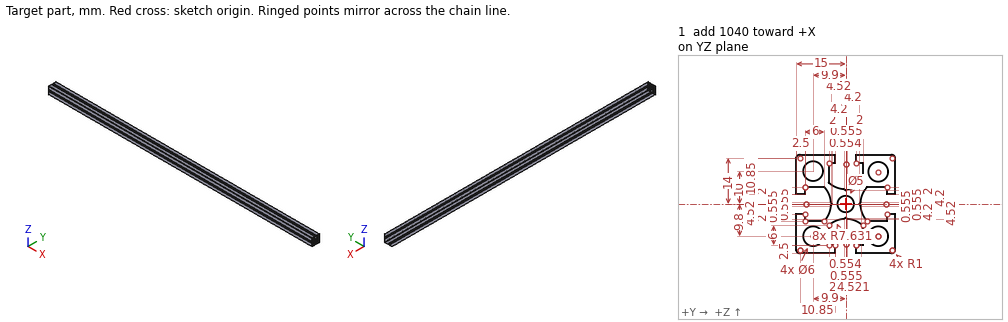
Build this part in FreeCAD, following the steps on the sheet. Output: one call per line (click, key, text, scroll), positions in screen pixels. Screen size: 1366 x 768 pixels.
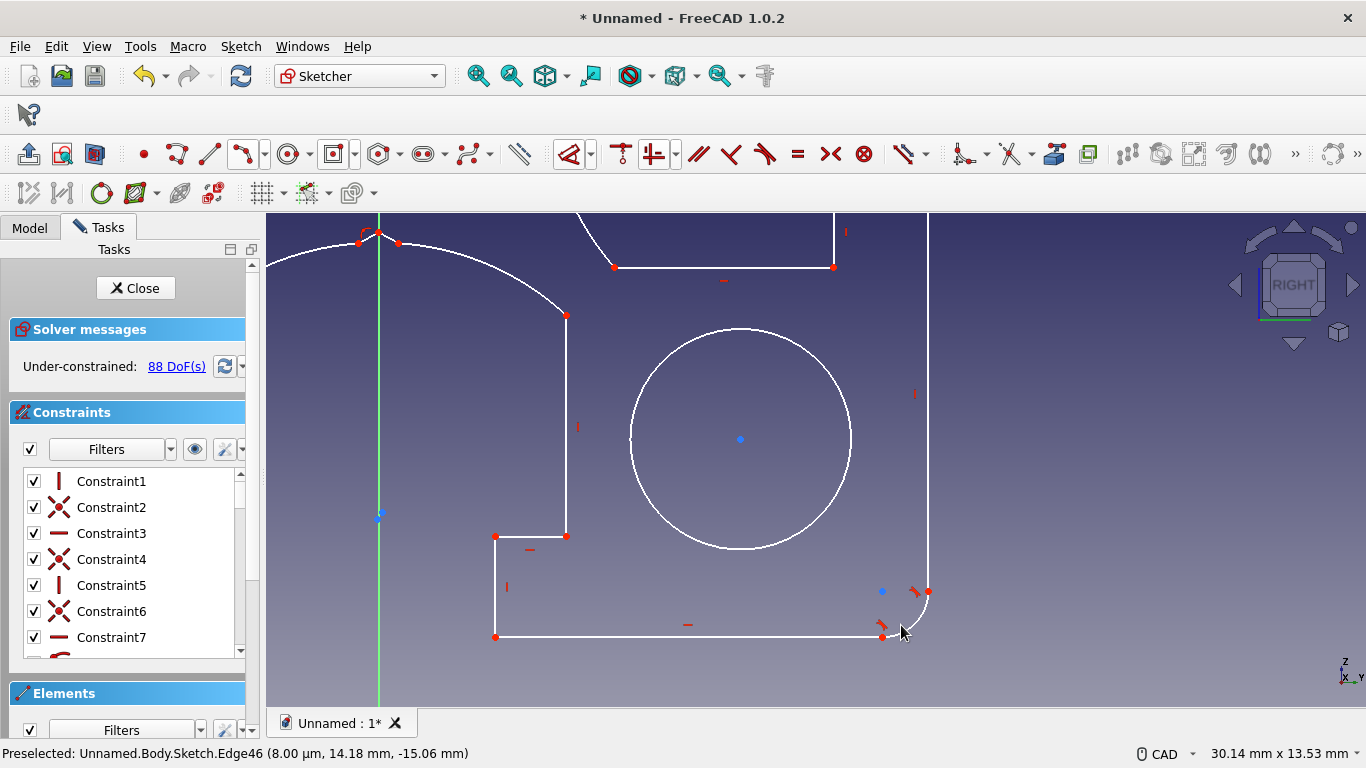
scroll(906, 625, down, 6)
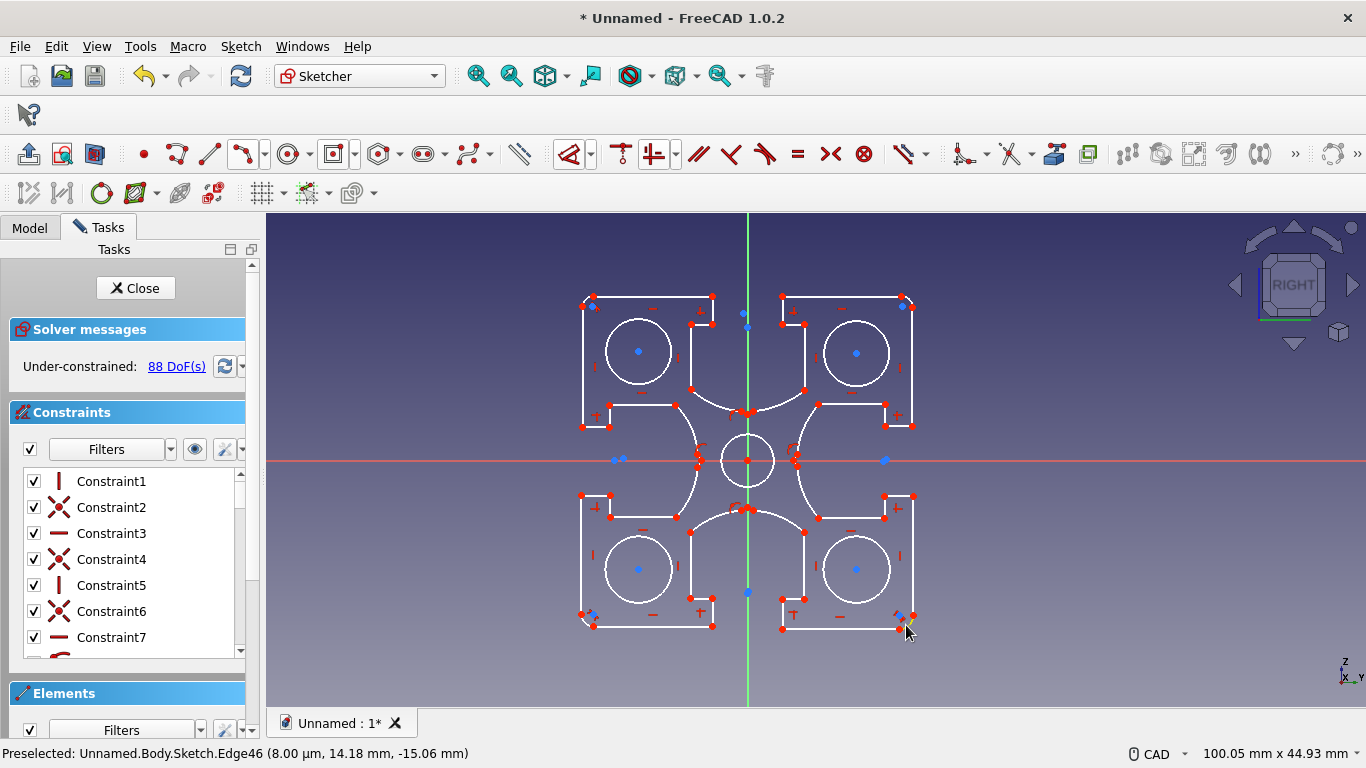
click(912, 391)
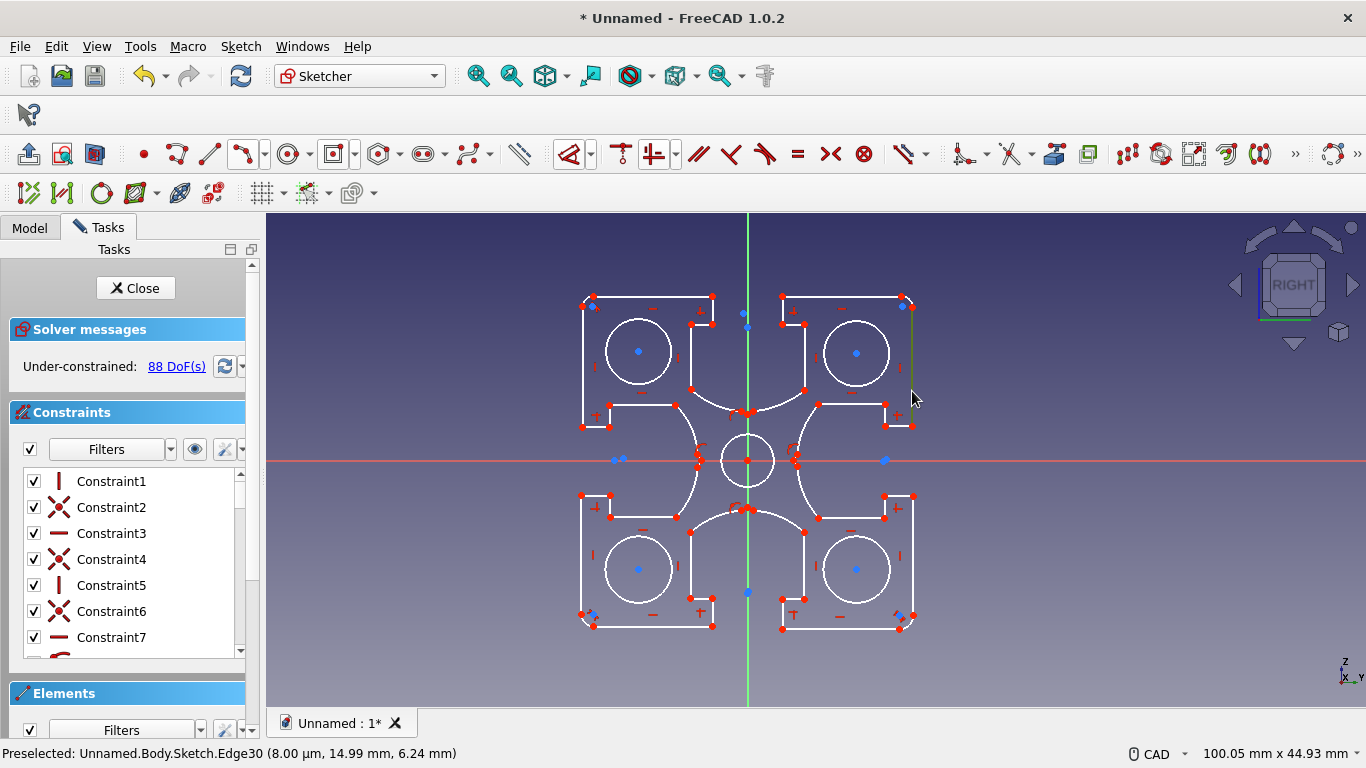
scroll(910, 300, up, 3)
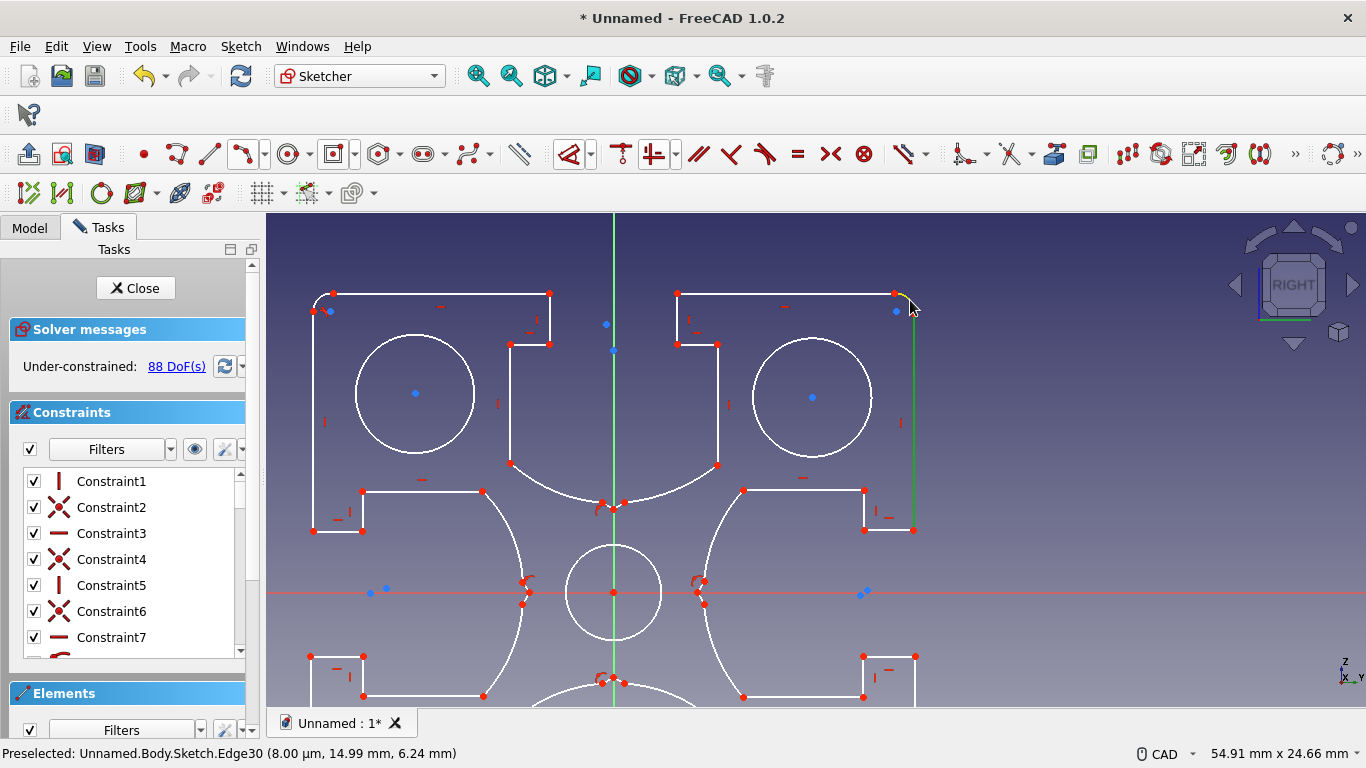
click(909, 299)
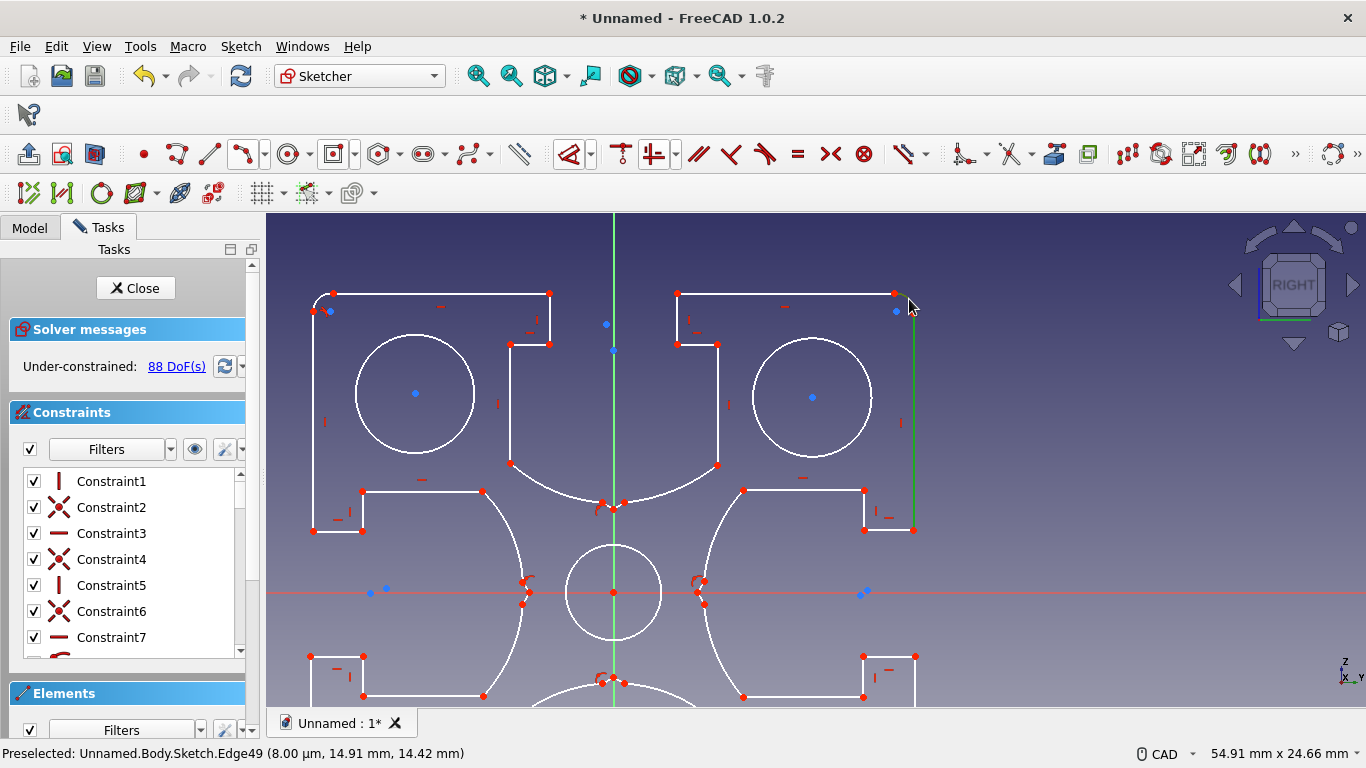
key(t)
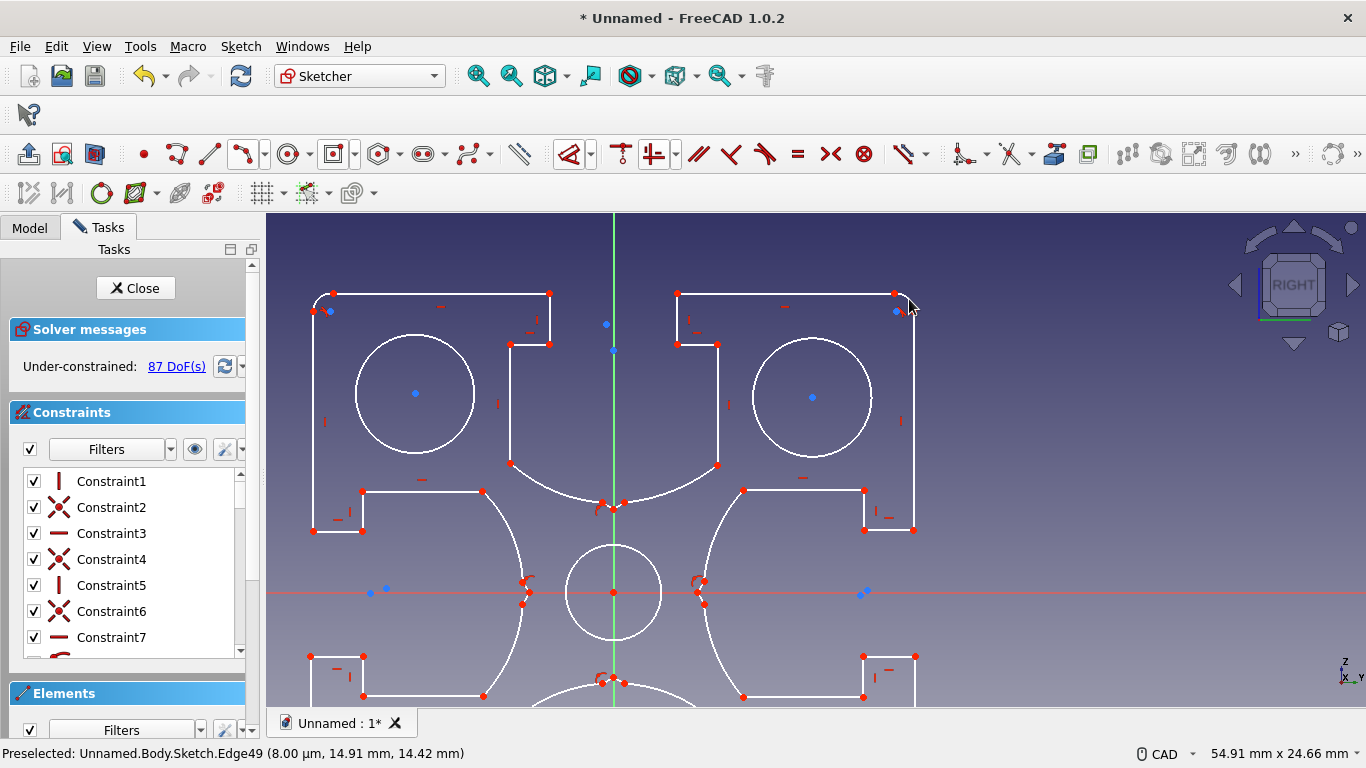
click(829, 294)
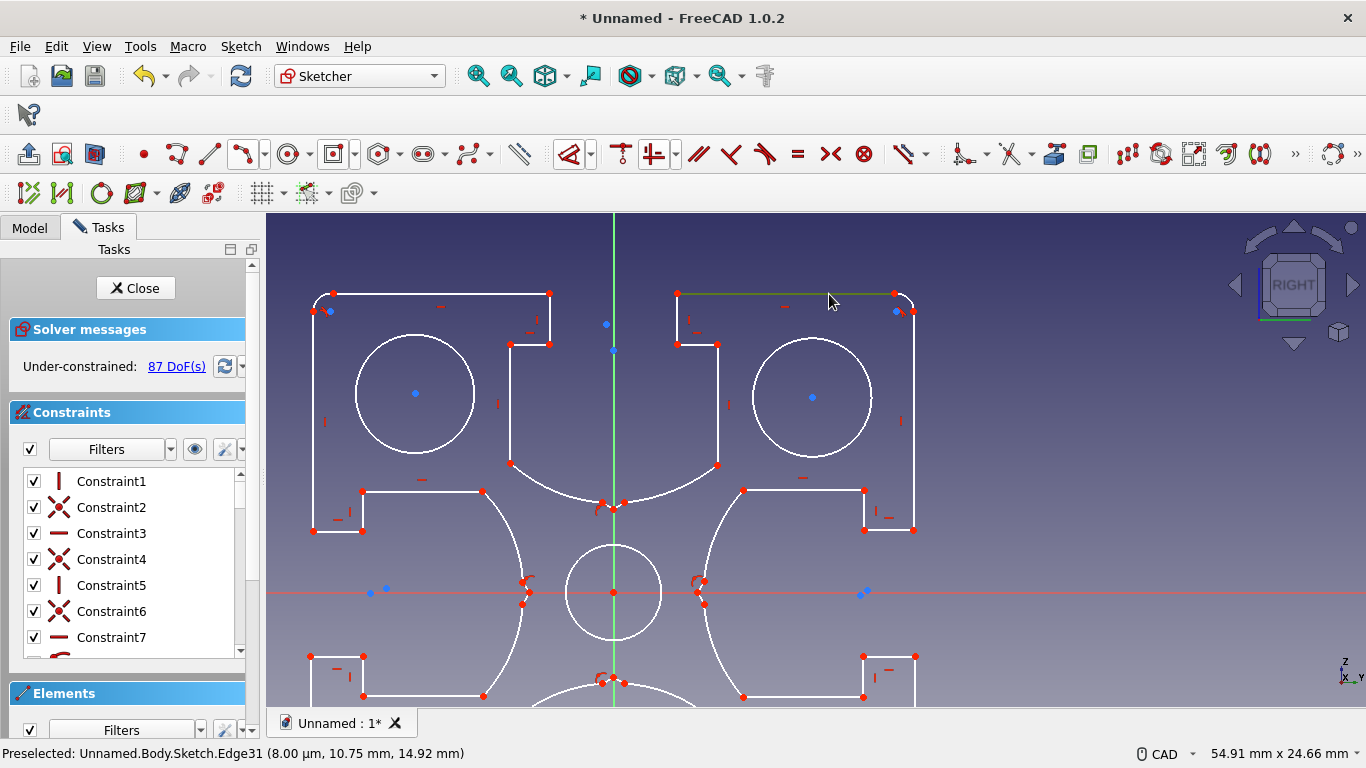
click(908, 298)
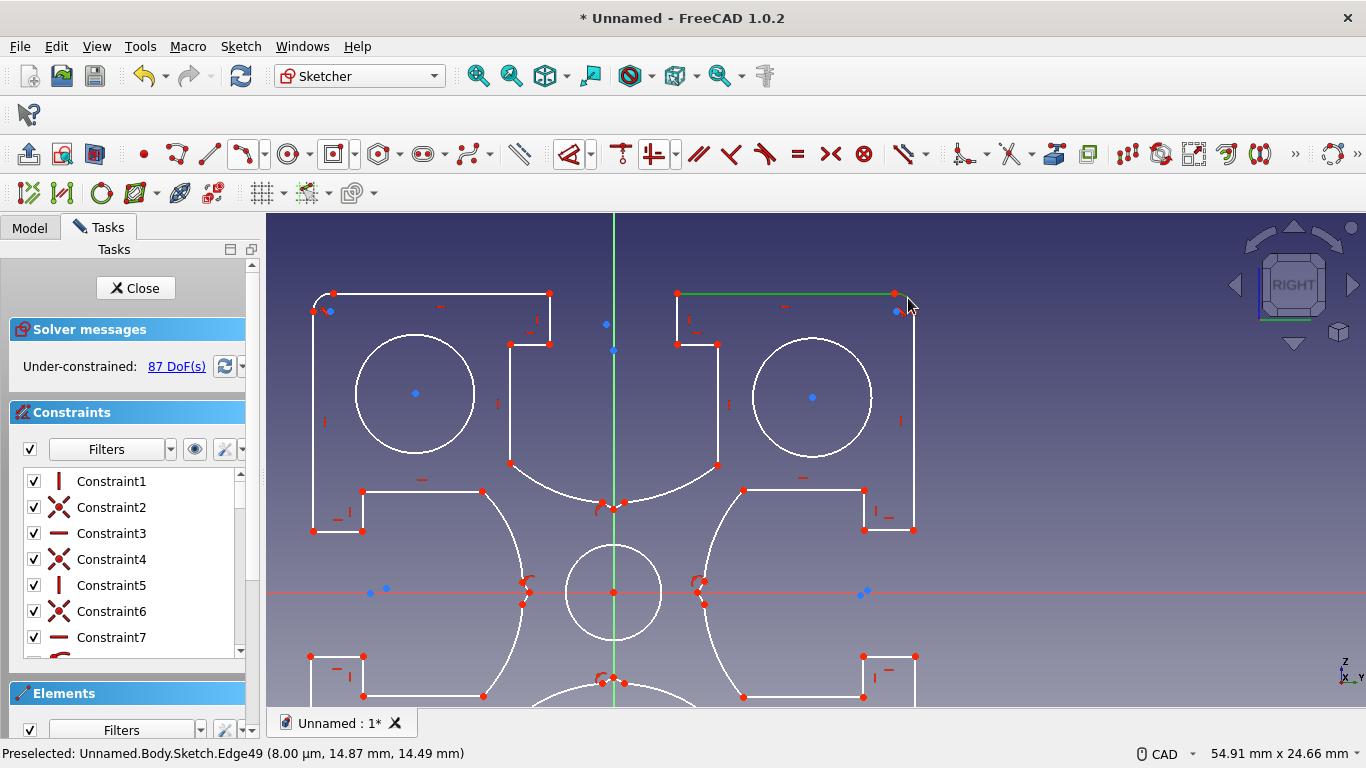
key(t)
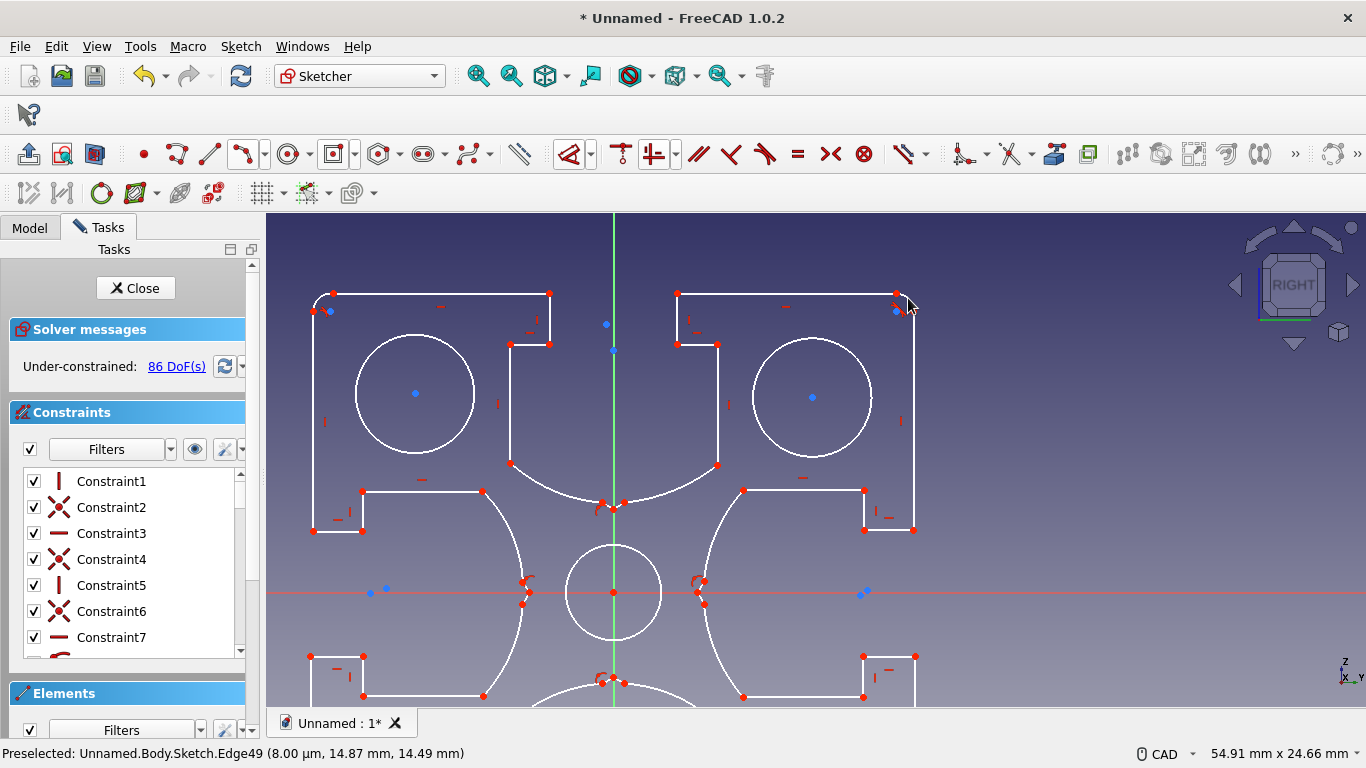
click(485, 294)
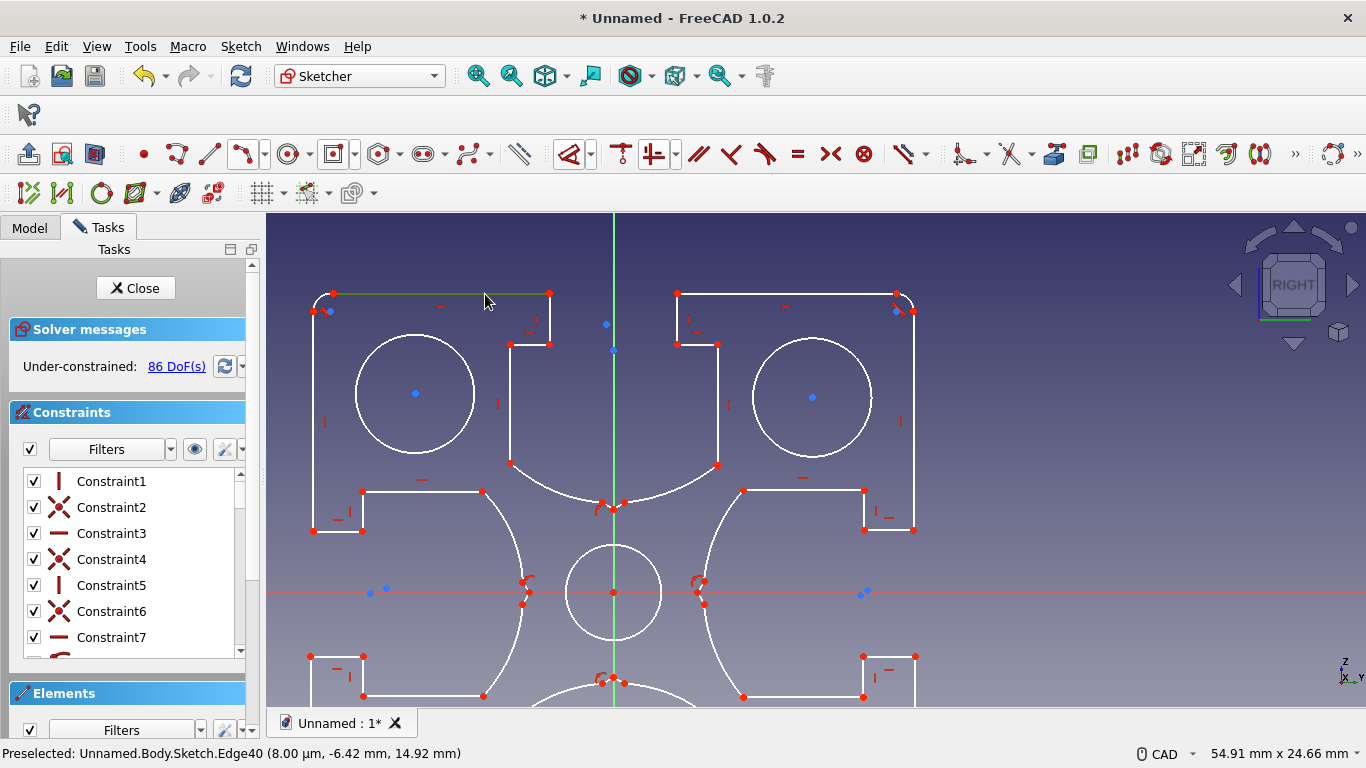
click(319, 298)